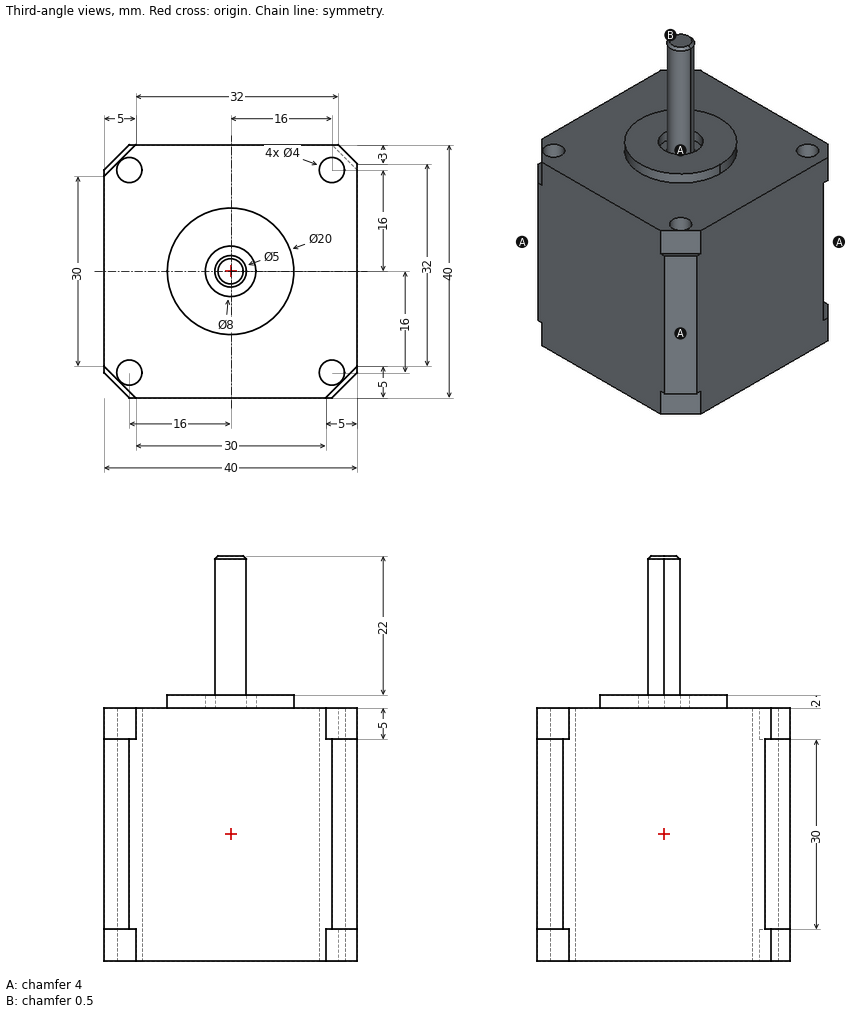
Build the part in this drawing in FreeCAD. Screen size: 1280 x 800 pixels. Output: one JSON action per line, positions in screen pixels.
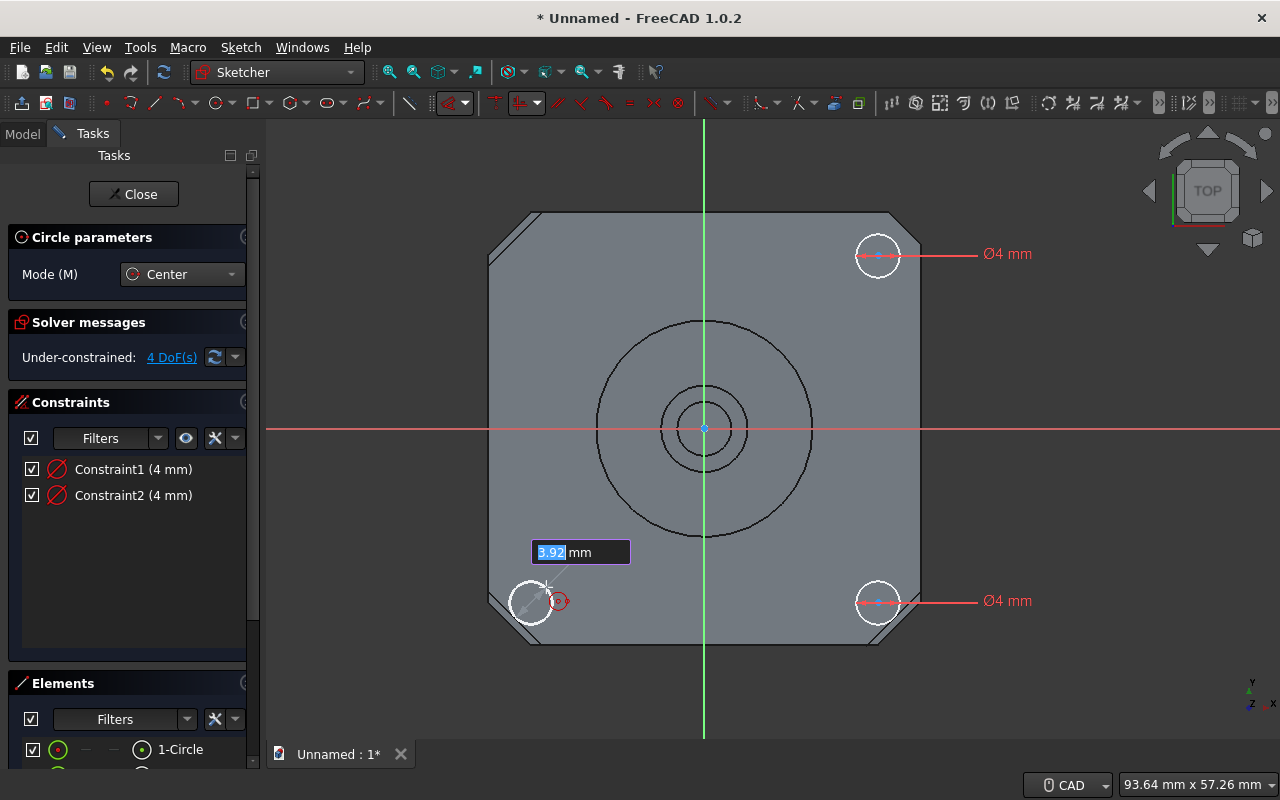
{"action": "type", "text": "4"}
{"action": "key", "text": "Return"}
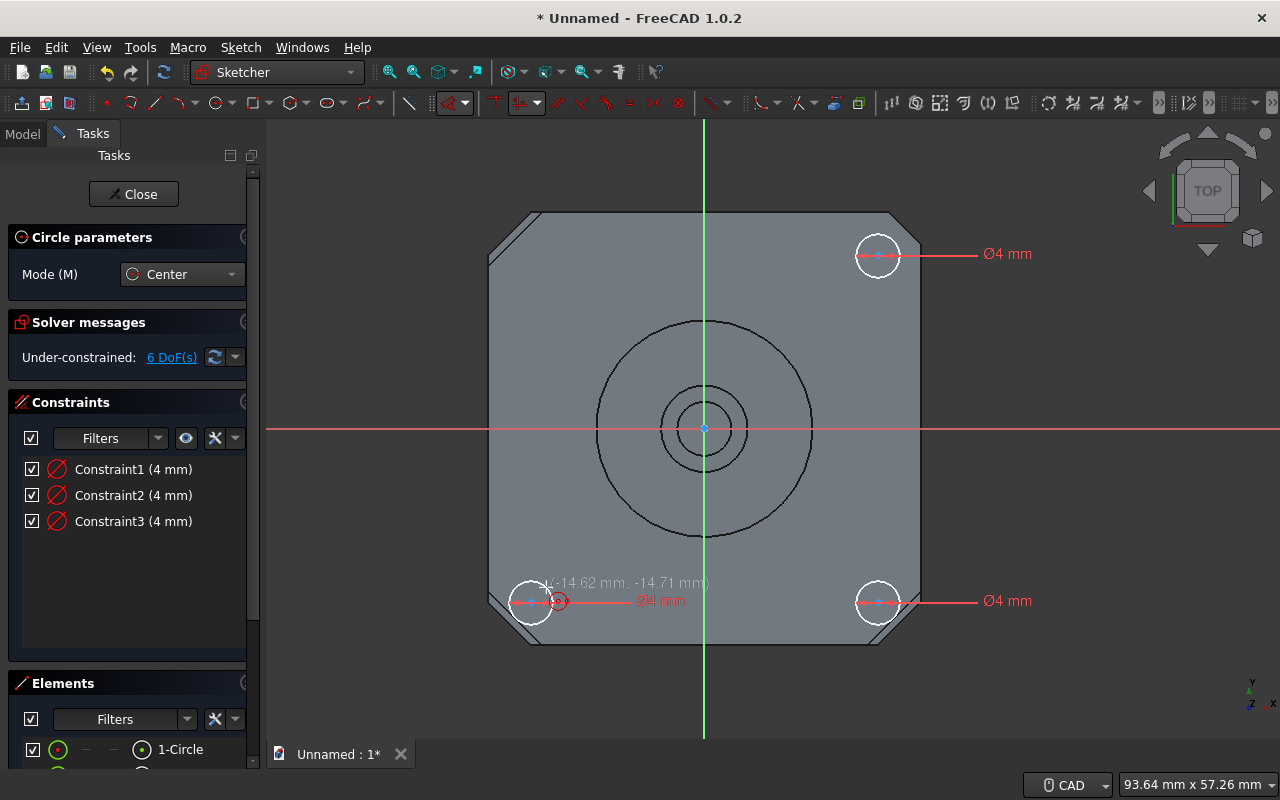
{"action": "left_click", "coordinate": [531, 255]}
{"action": "mouse_move", "coordinate": [546, 240]}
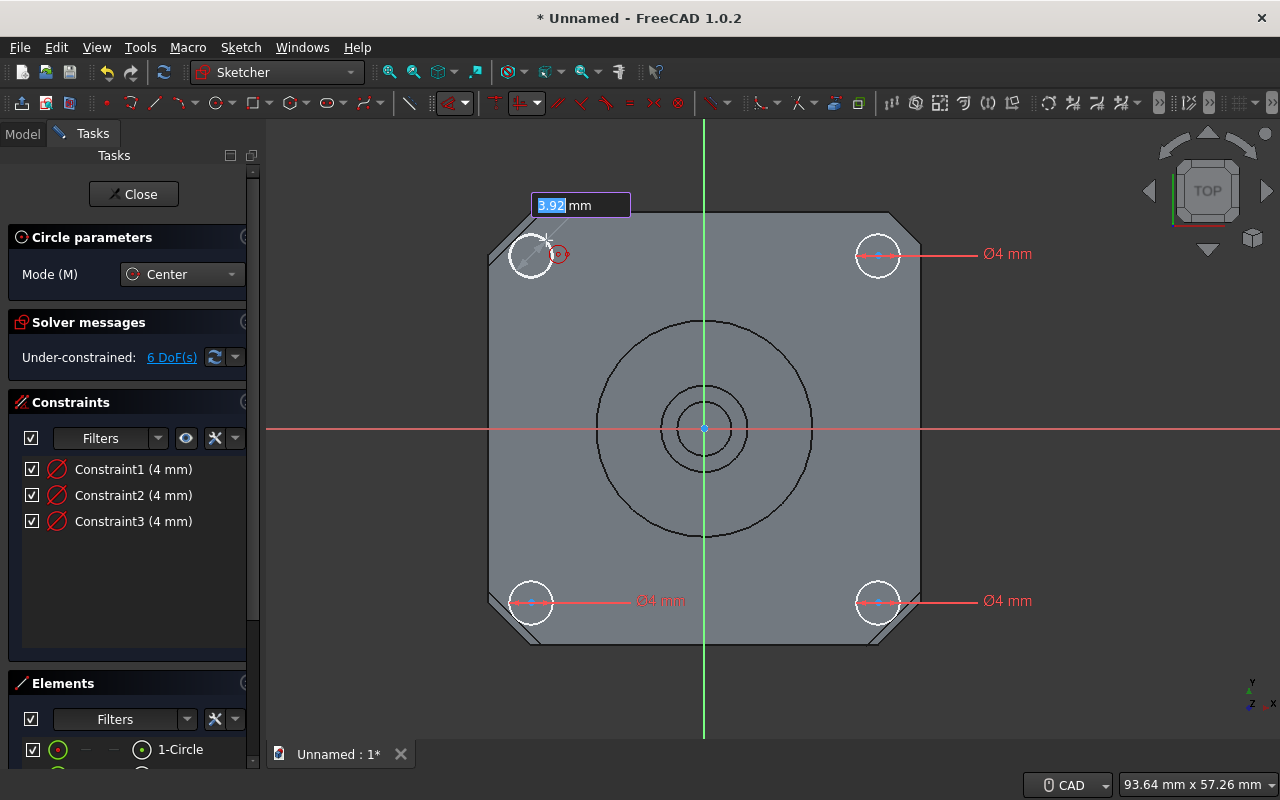
{"action": "type", "text": "4"}
{"action": "key", "text": "Return"}
{"action": "key", "text": "Escape"}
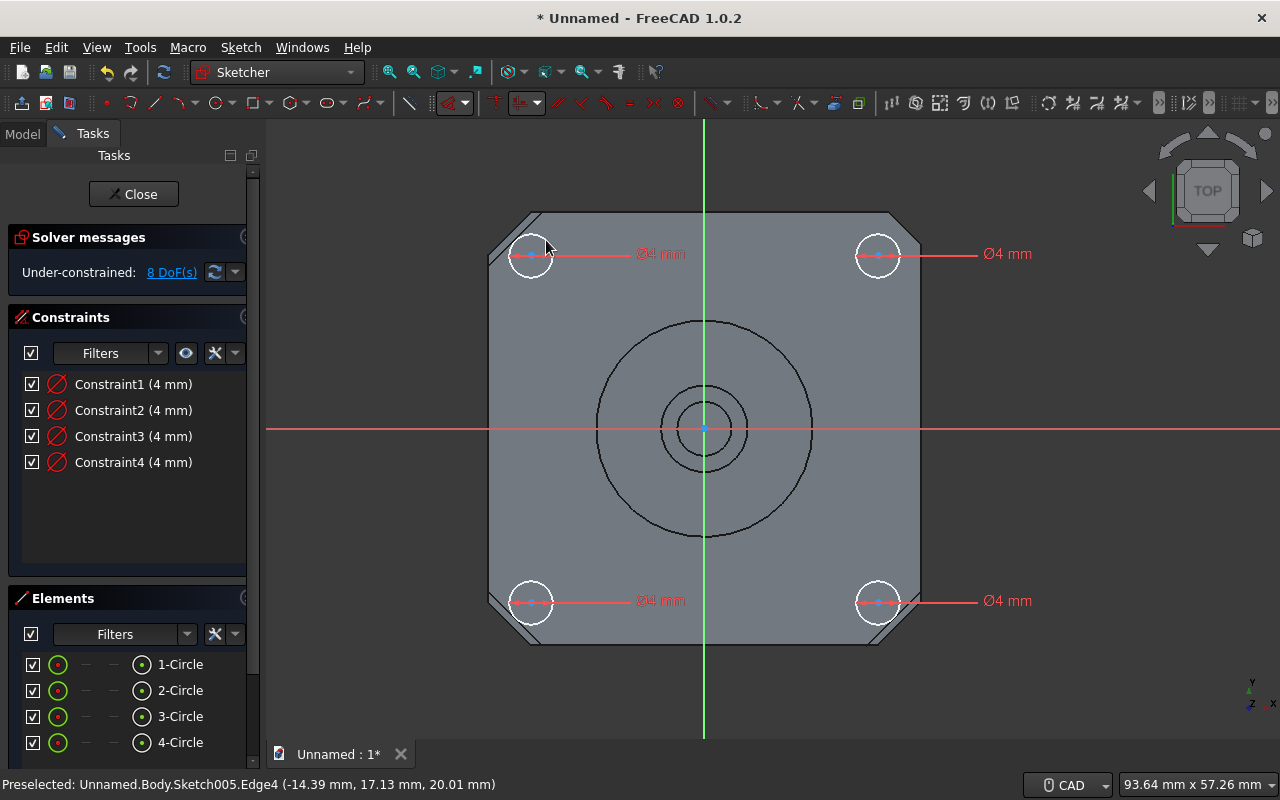
{"action": "left_click", "coordinate": [878, 256]}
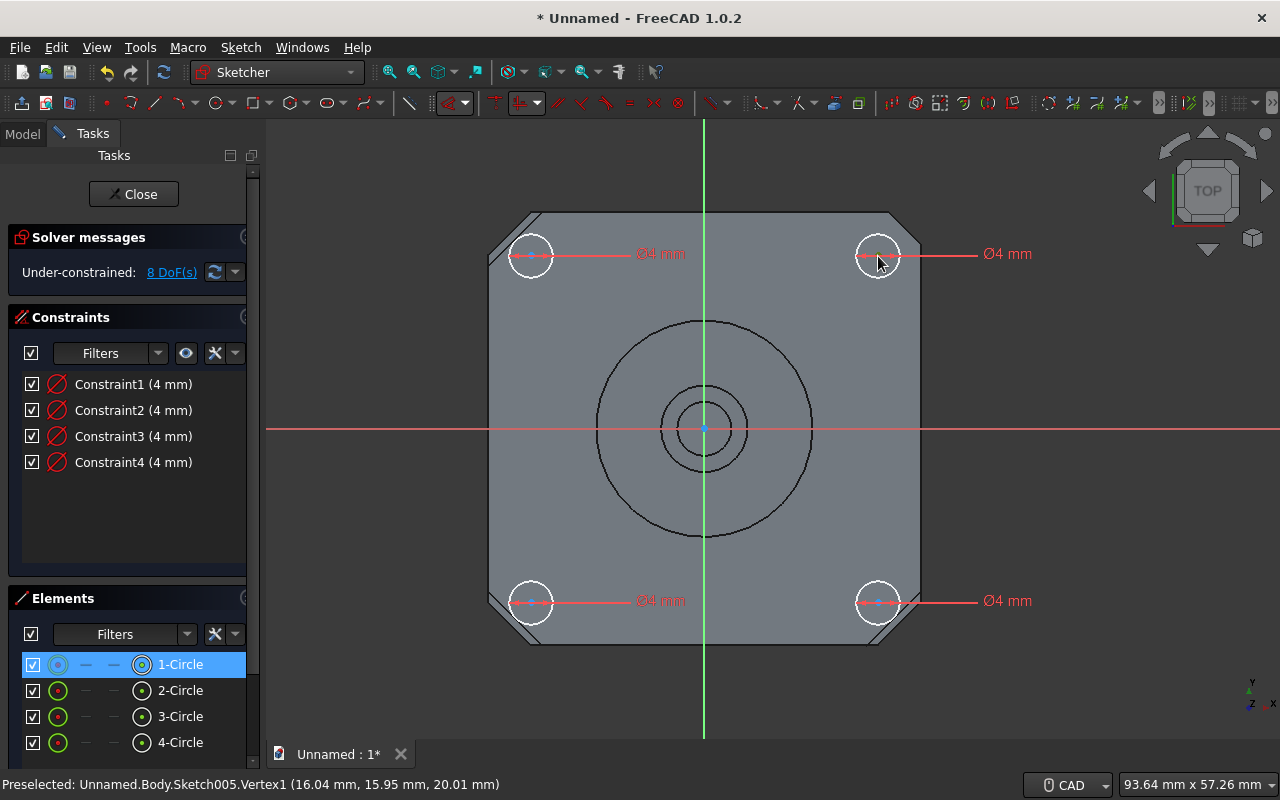
{"action": "left_click", "coordinate": [878, 603]}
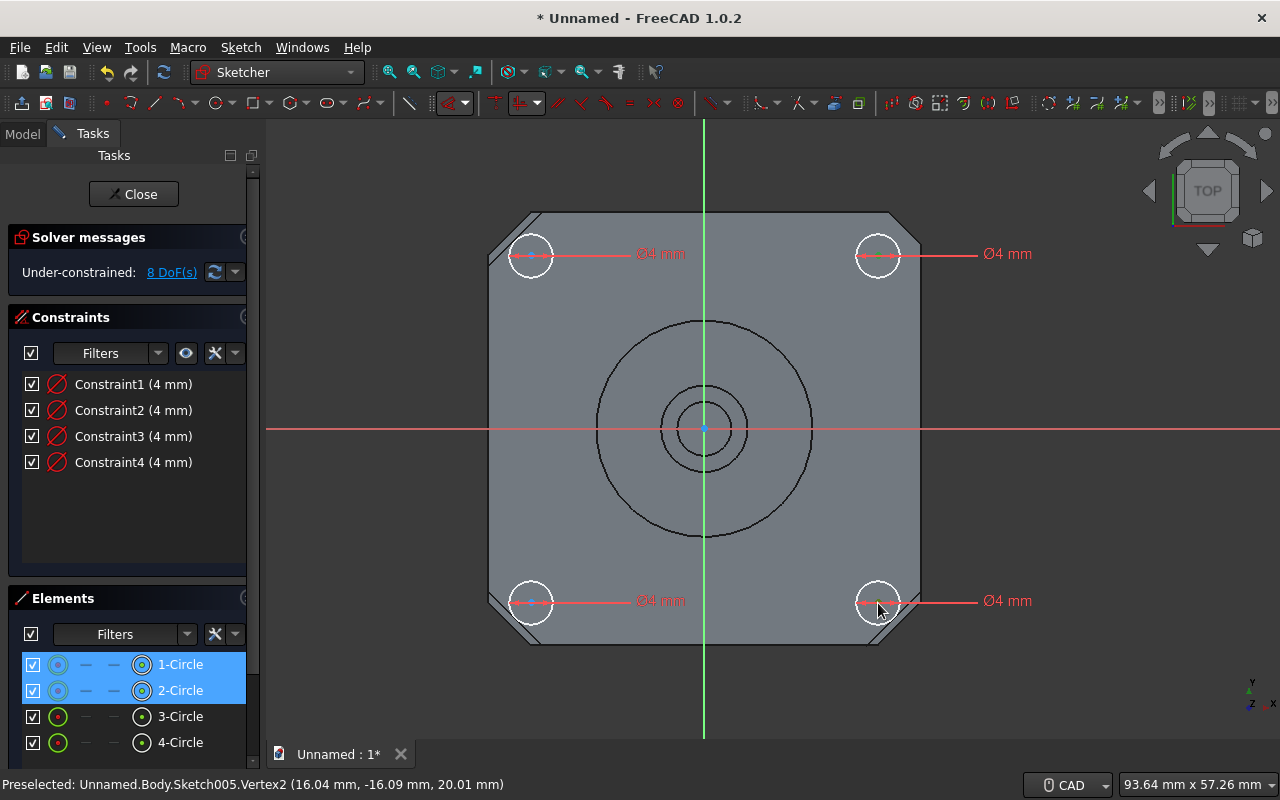
{"action": "left_click", "coordinate": [540, 104]}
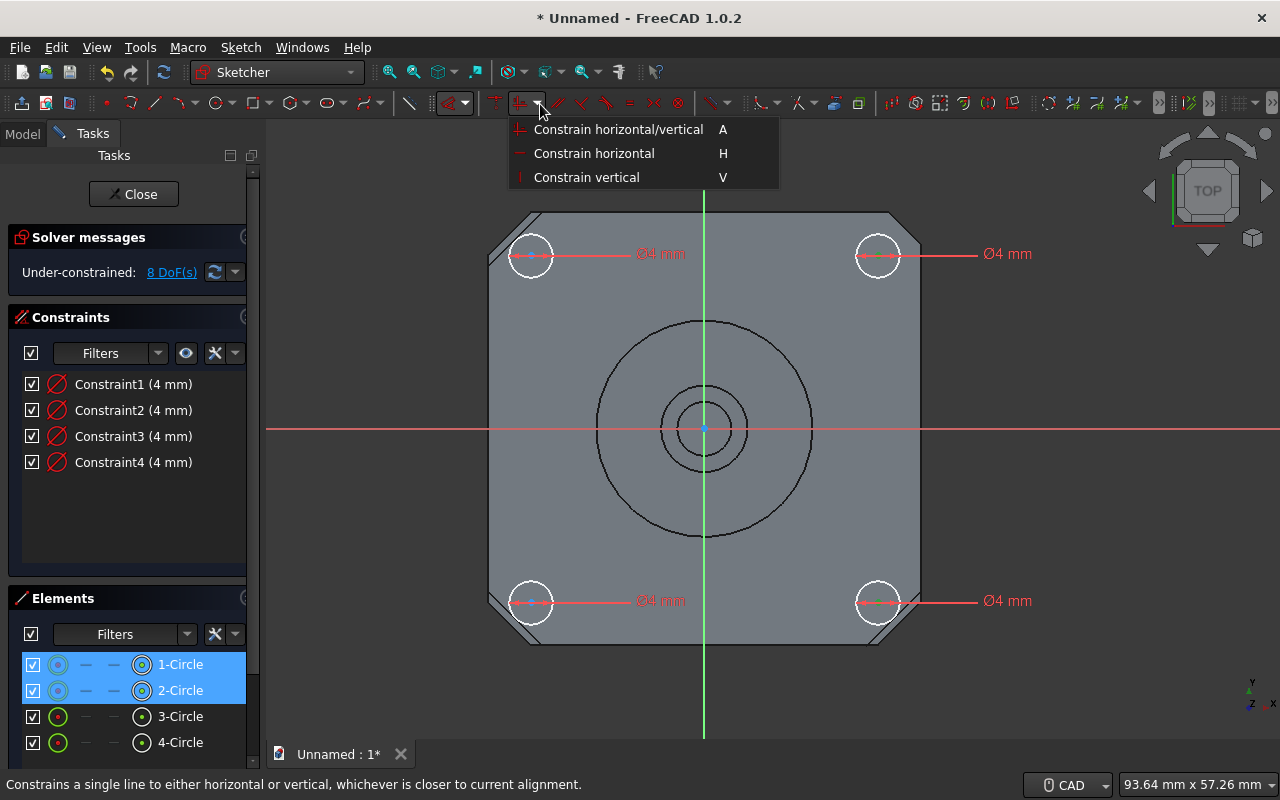
{"action": "left_click", "coordinate": [644, 177]}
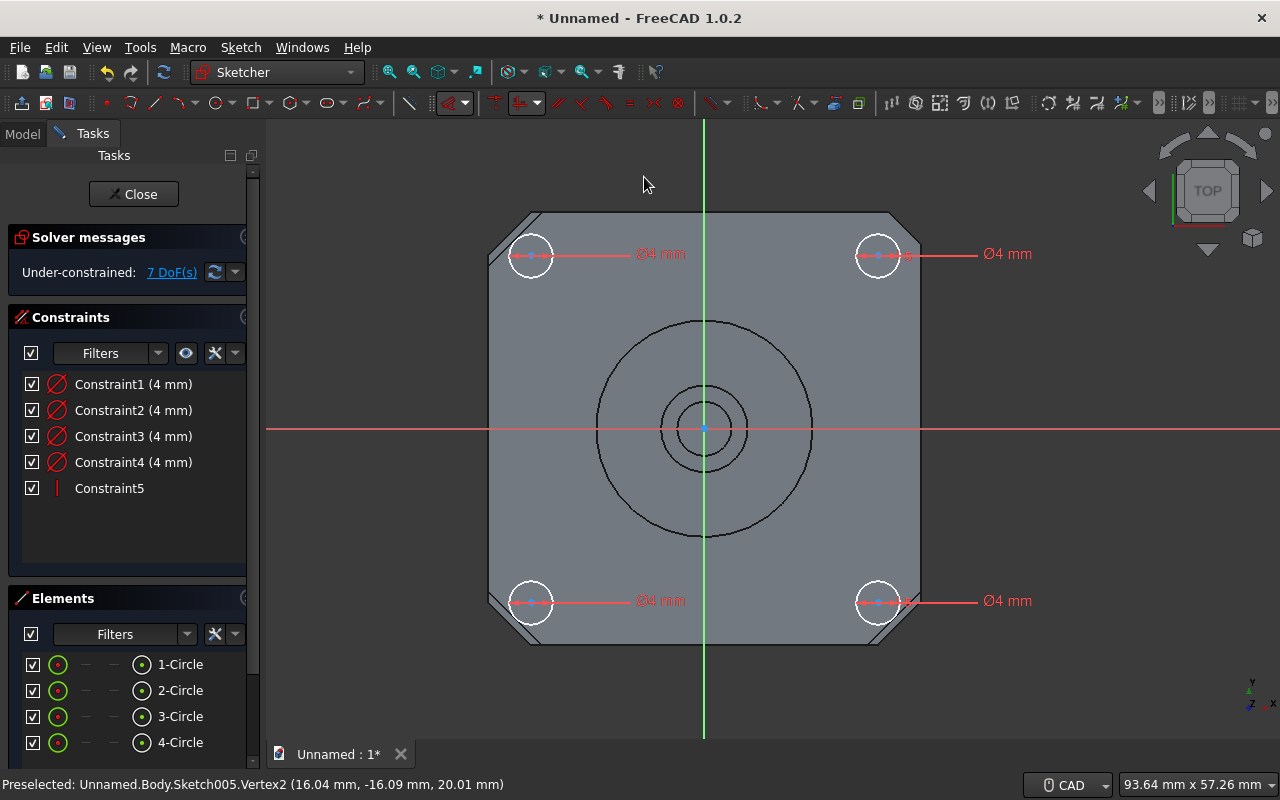
{"action": "left_click", "coordinate": [878, 603]}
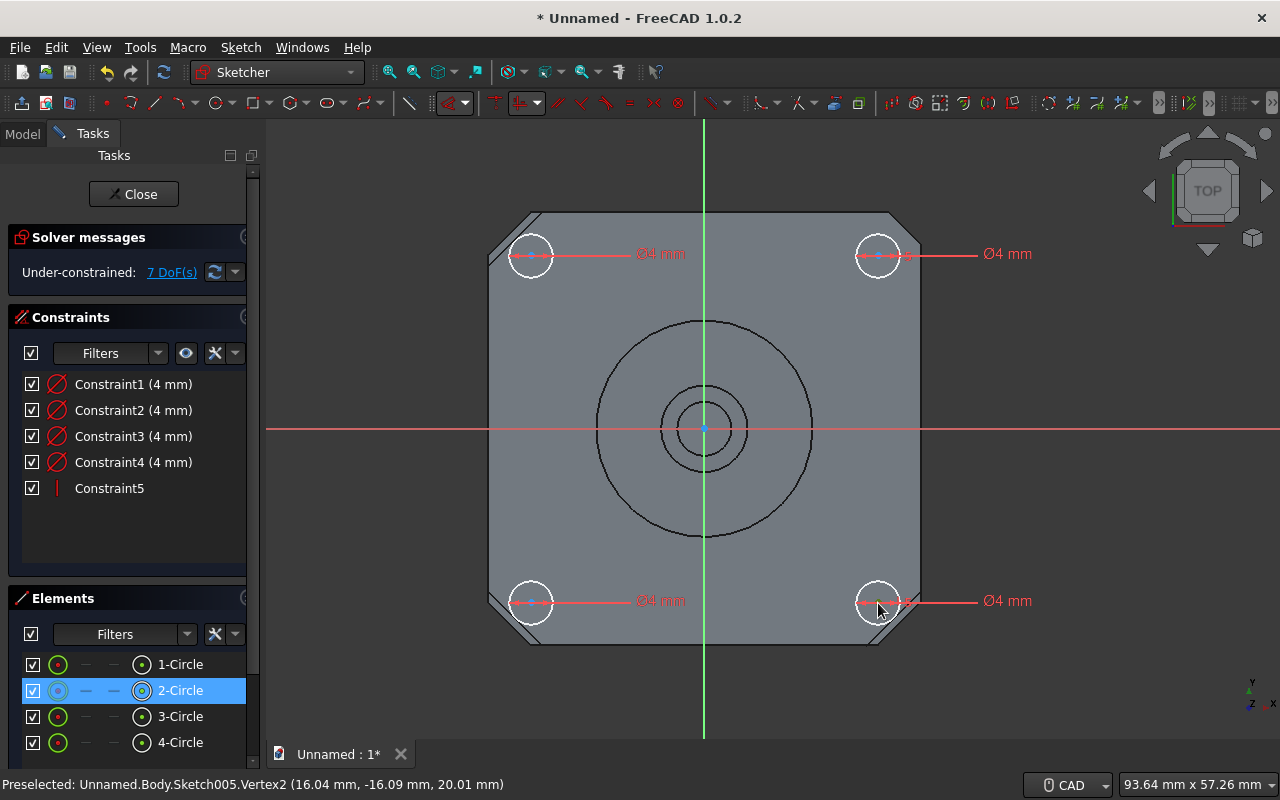
{"action": "left_click", "coordinate": [531, 603]}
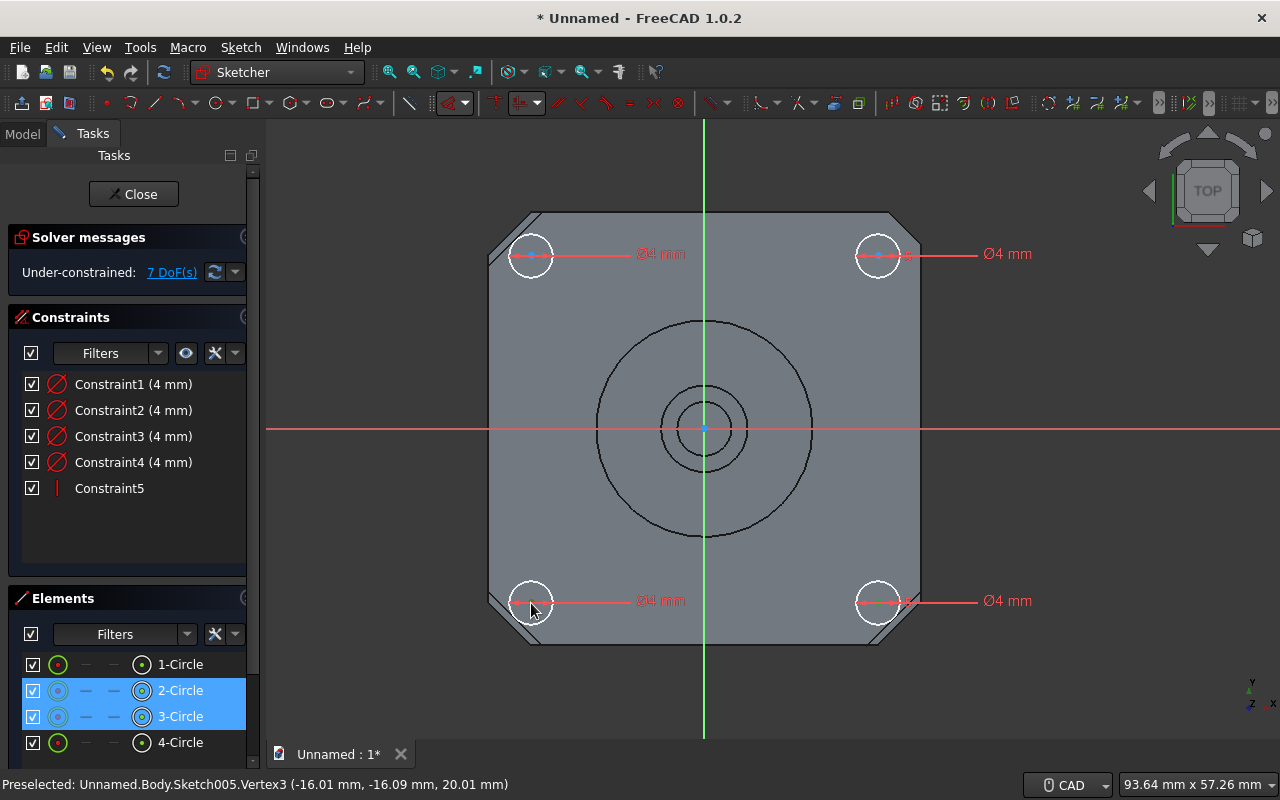
{"action": "left_click", "coordinate": [540, 104]}